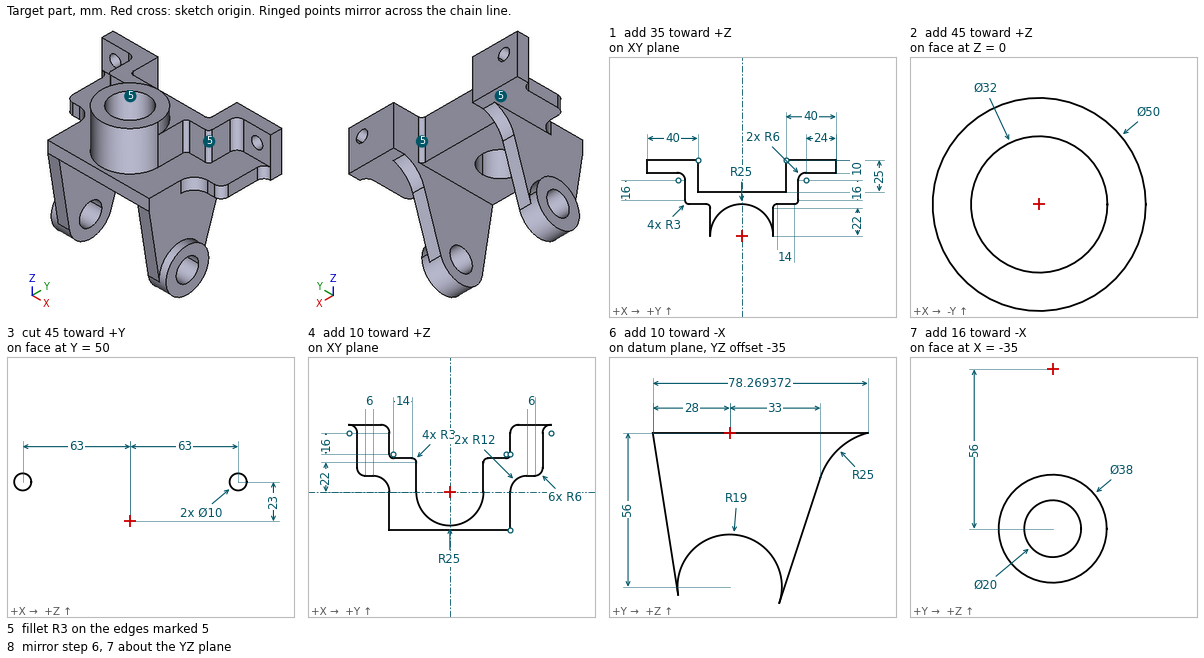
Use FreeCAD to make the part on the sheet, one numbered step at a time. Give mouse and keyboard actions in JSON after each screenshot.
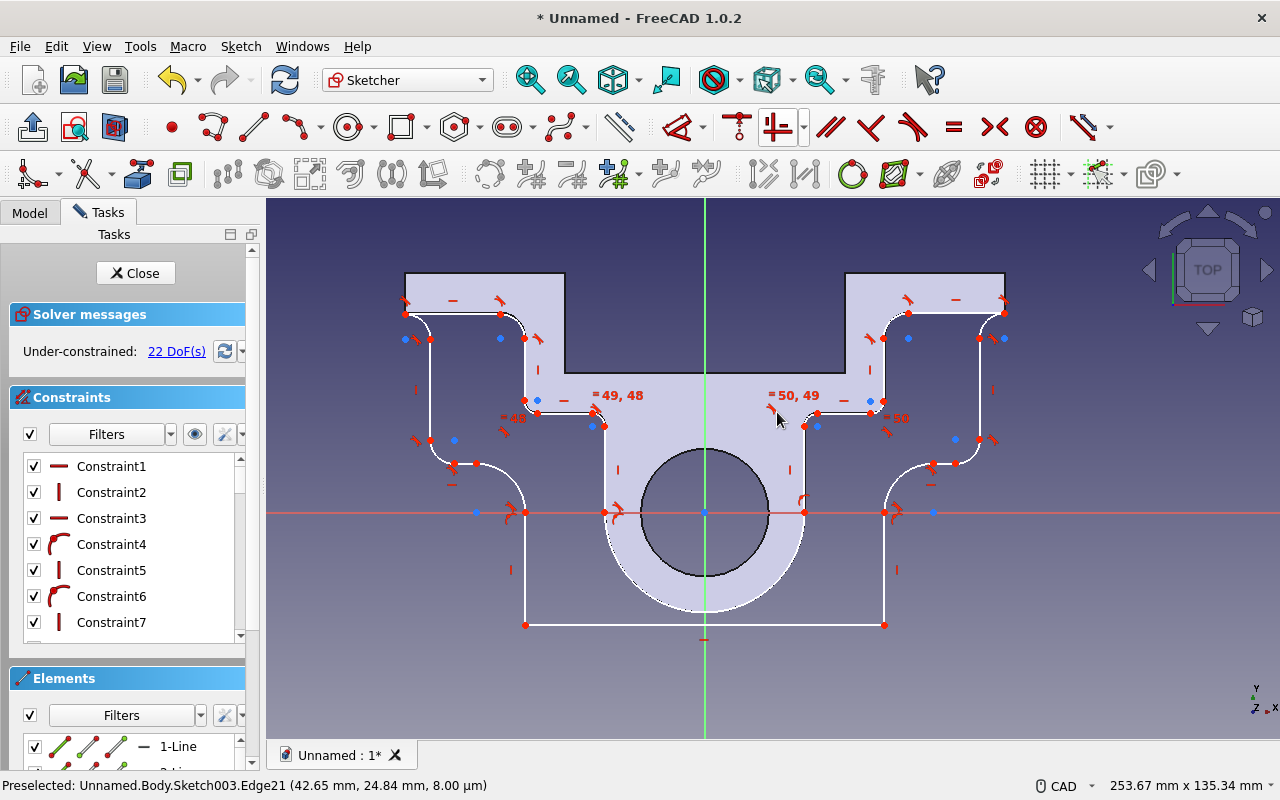
{"action": "scroll", "coordinate": [522, 327], "scroll_direction": "up", "scroll_amount": 2}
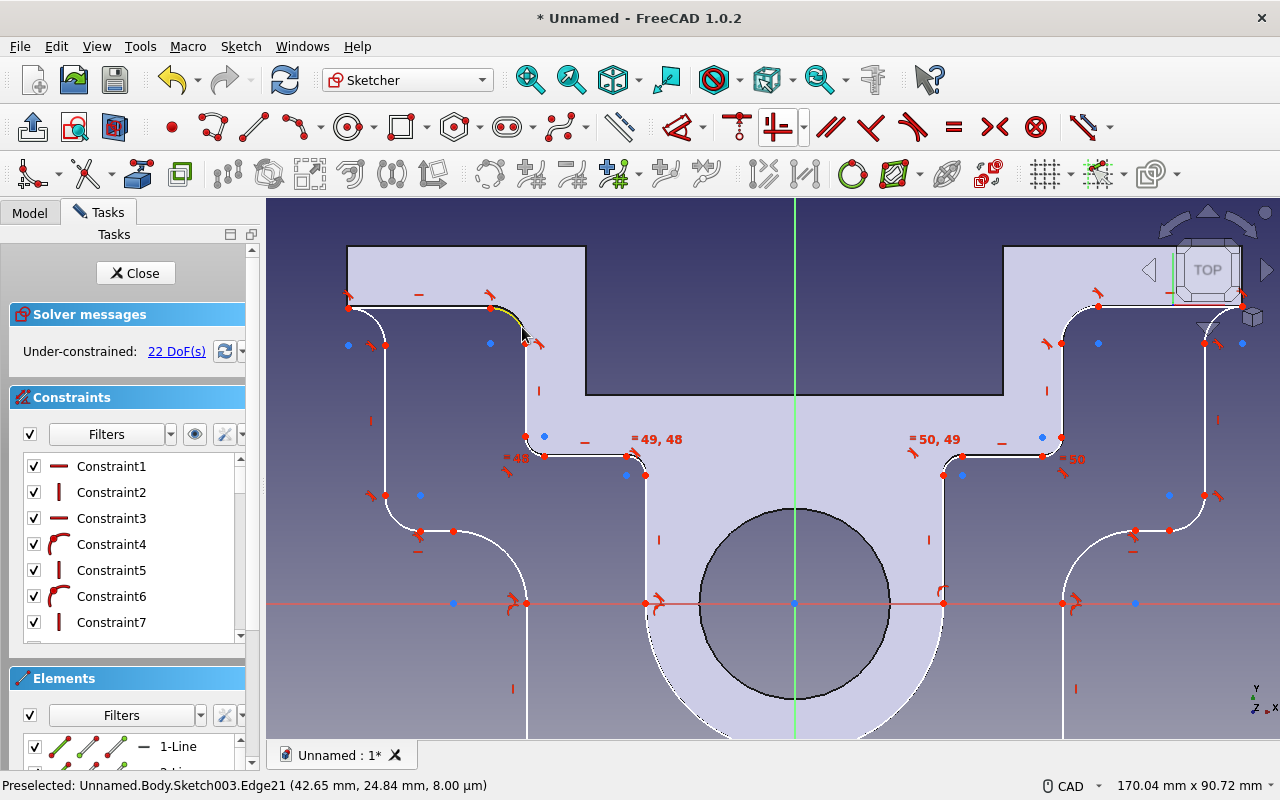
{"action": "left_click", "coordinate": [522, 328]}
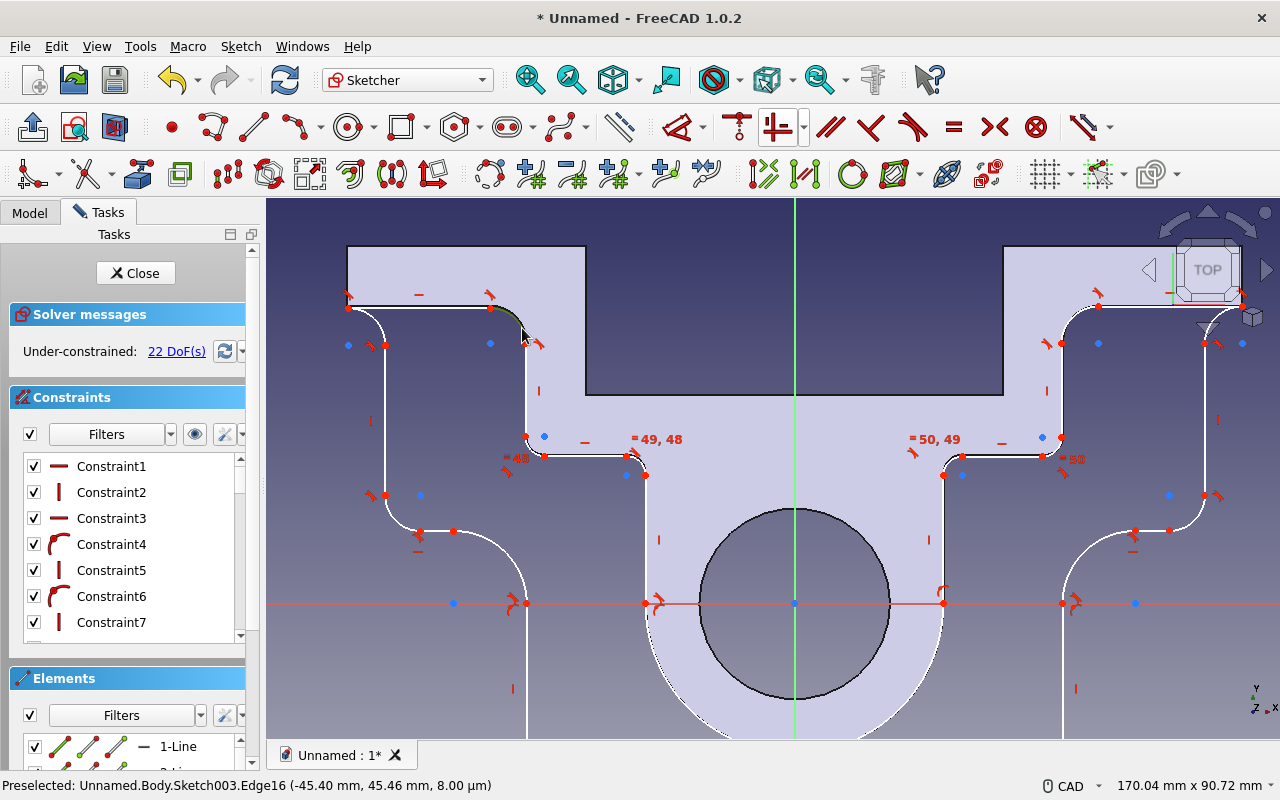
{"action": "left_click", "coordinate": [1082, 311]}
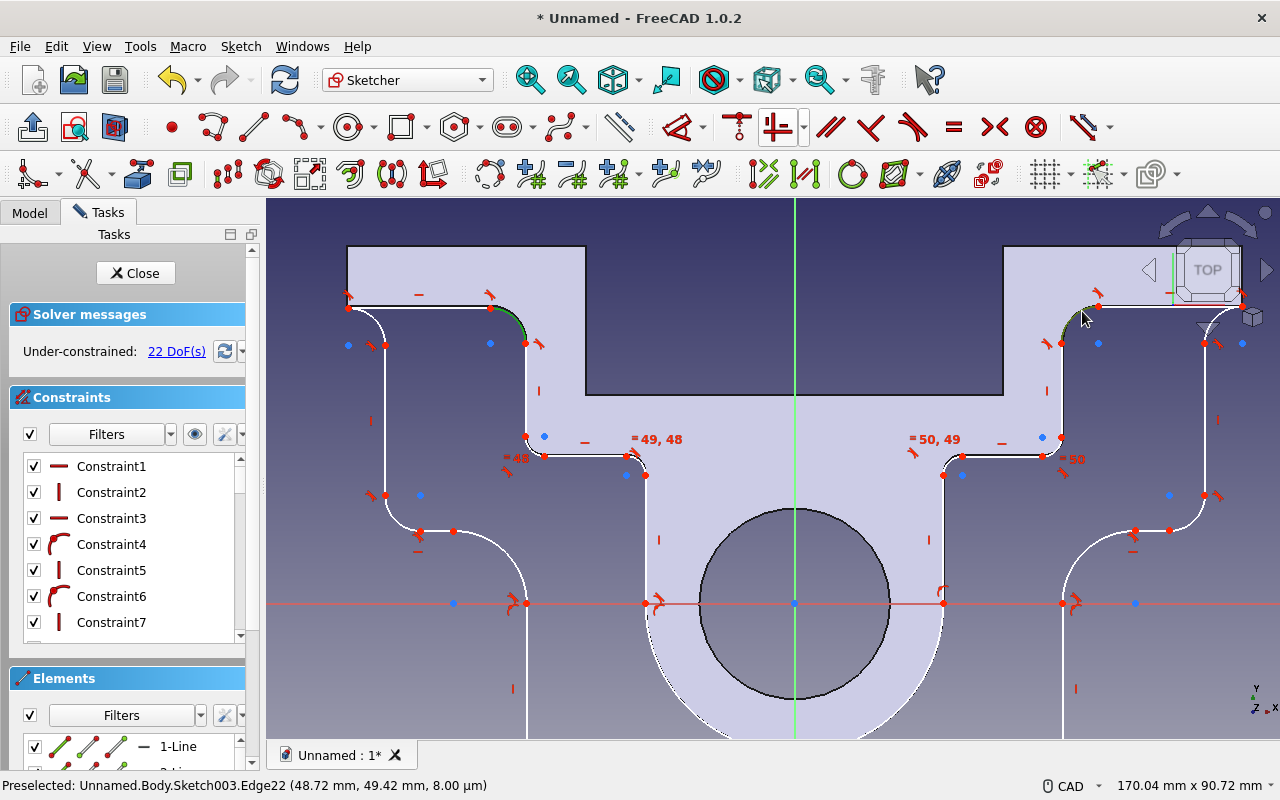
{"action": "scroll", "coordinate": [521, 327], "scroll_direction": "down", "scroll_amount": 2}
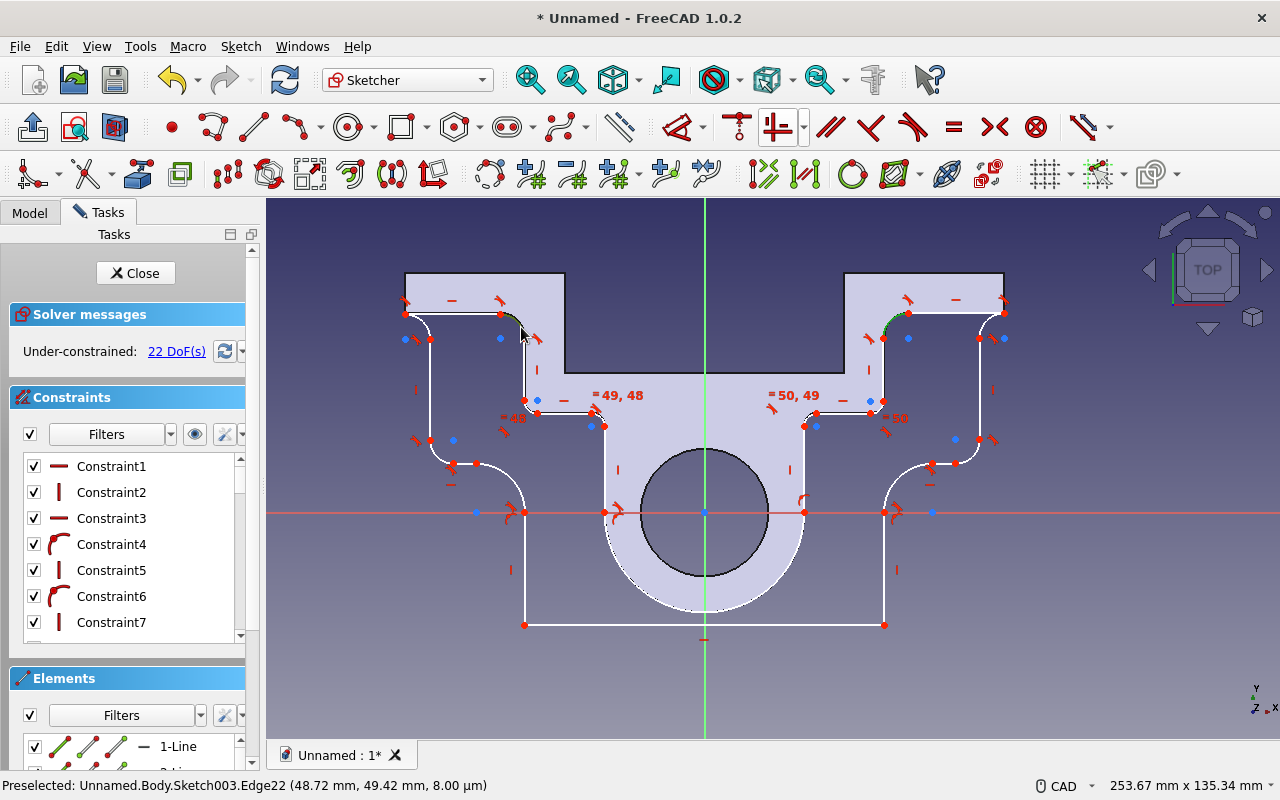
{"action": "left_click", "coordinate": [982, 327]}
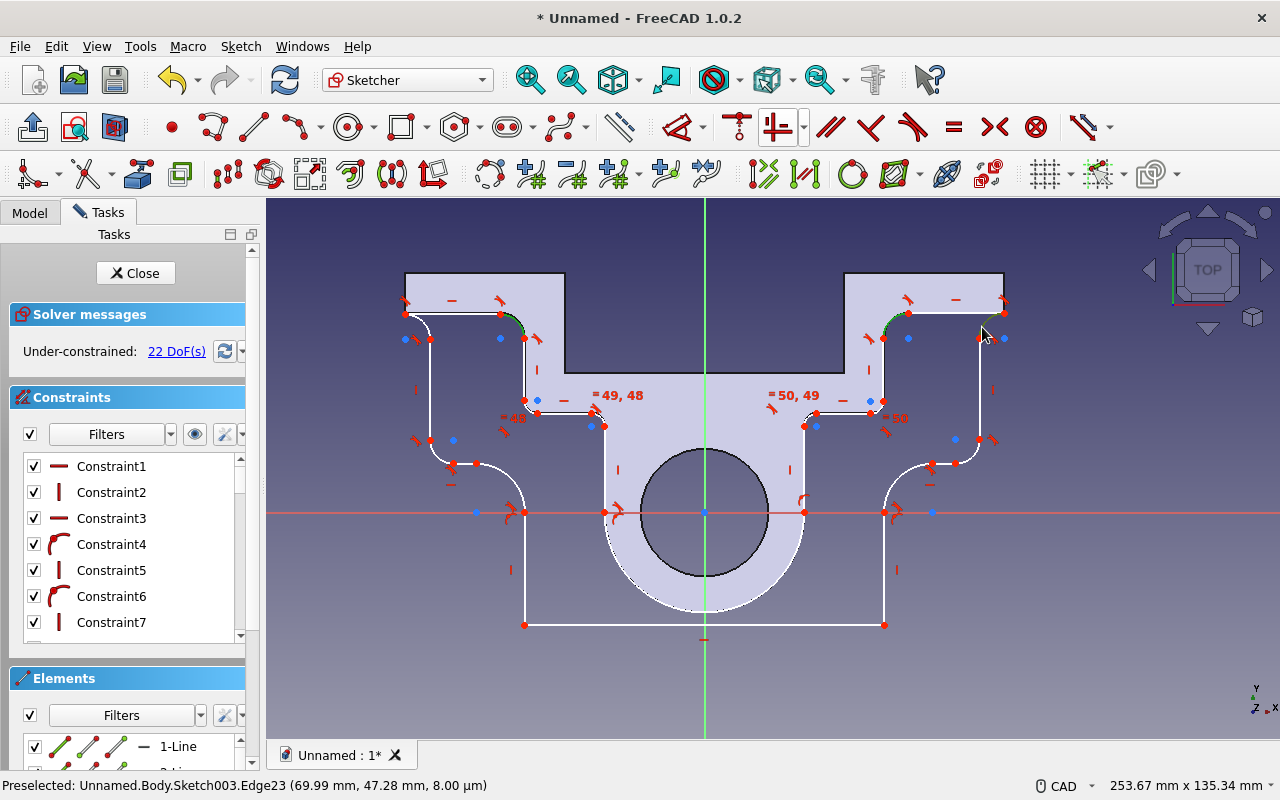
{"action": "scroll", "coordinate": [966, 461], "scroll_direction": "up", "scroll_amount": 2}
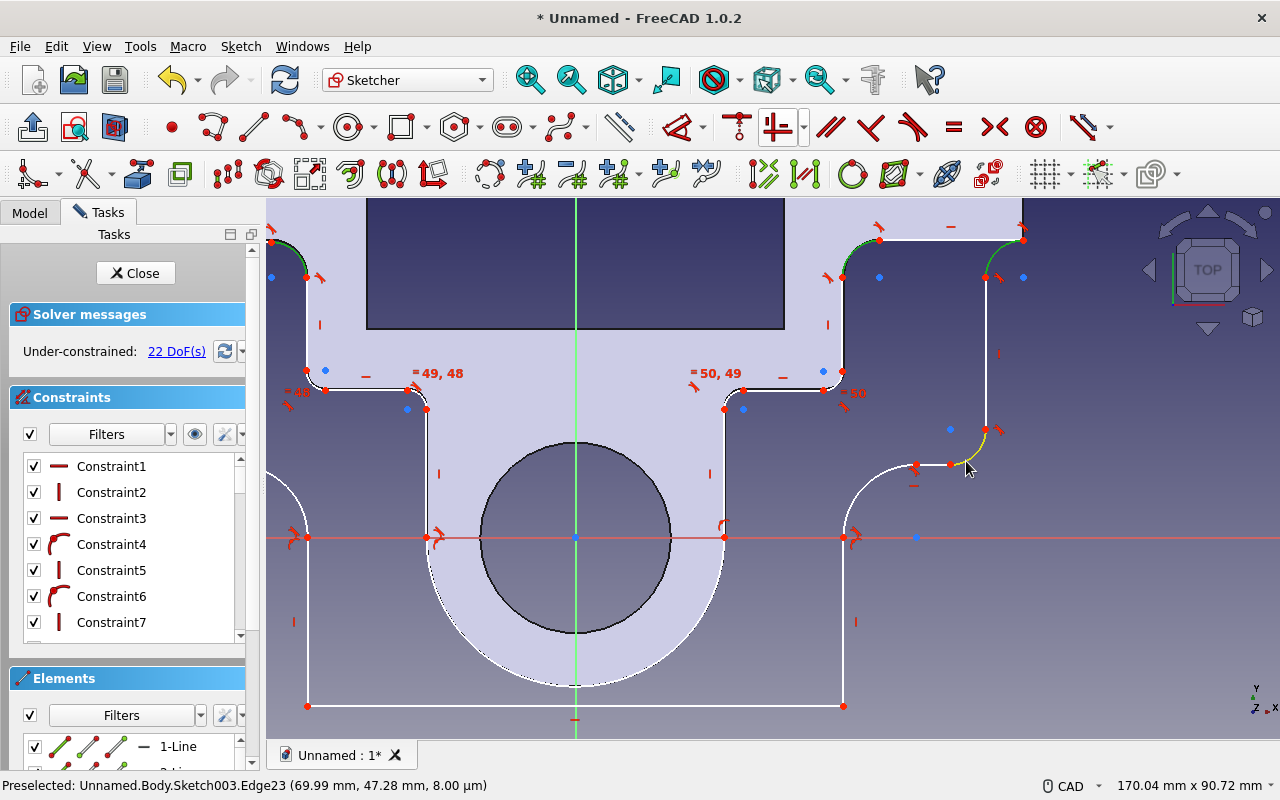
{"action": "left_click", "coordinate": [966, 461]}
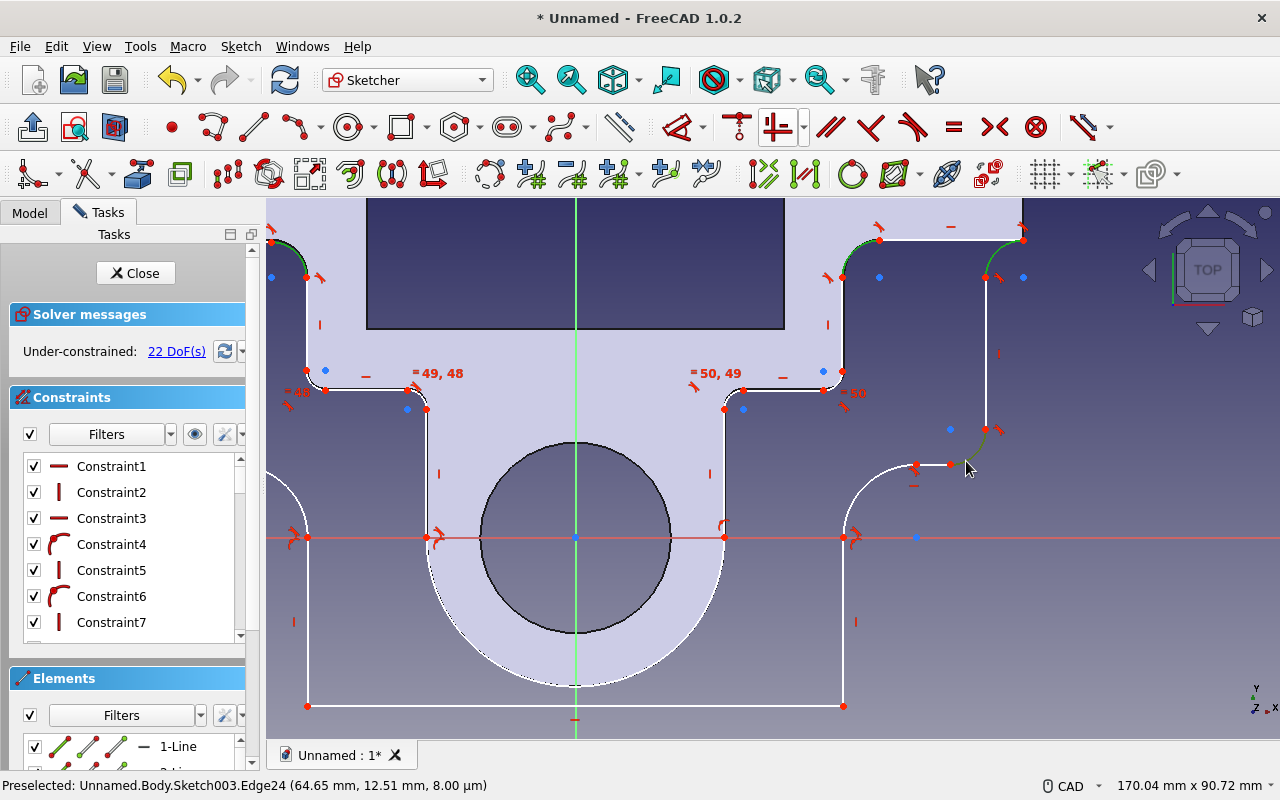
{"action": "scroll", "coordinate": [967, 461], "scroll_direction": "down", "scroll_amount": 2}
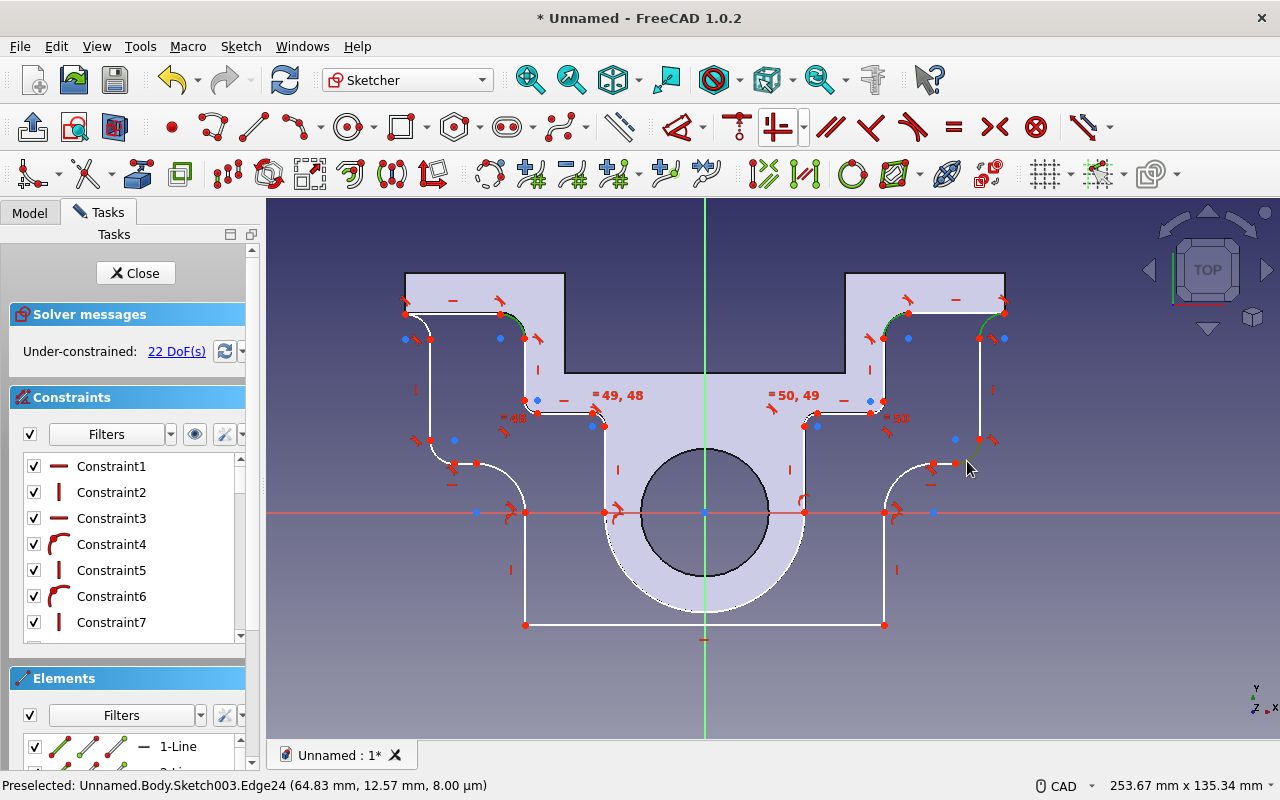
{"action": "scroll", "coordinate": [433, 451], "scroll_direction": "up", "scroll_amount": 2}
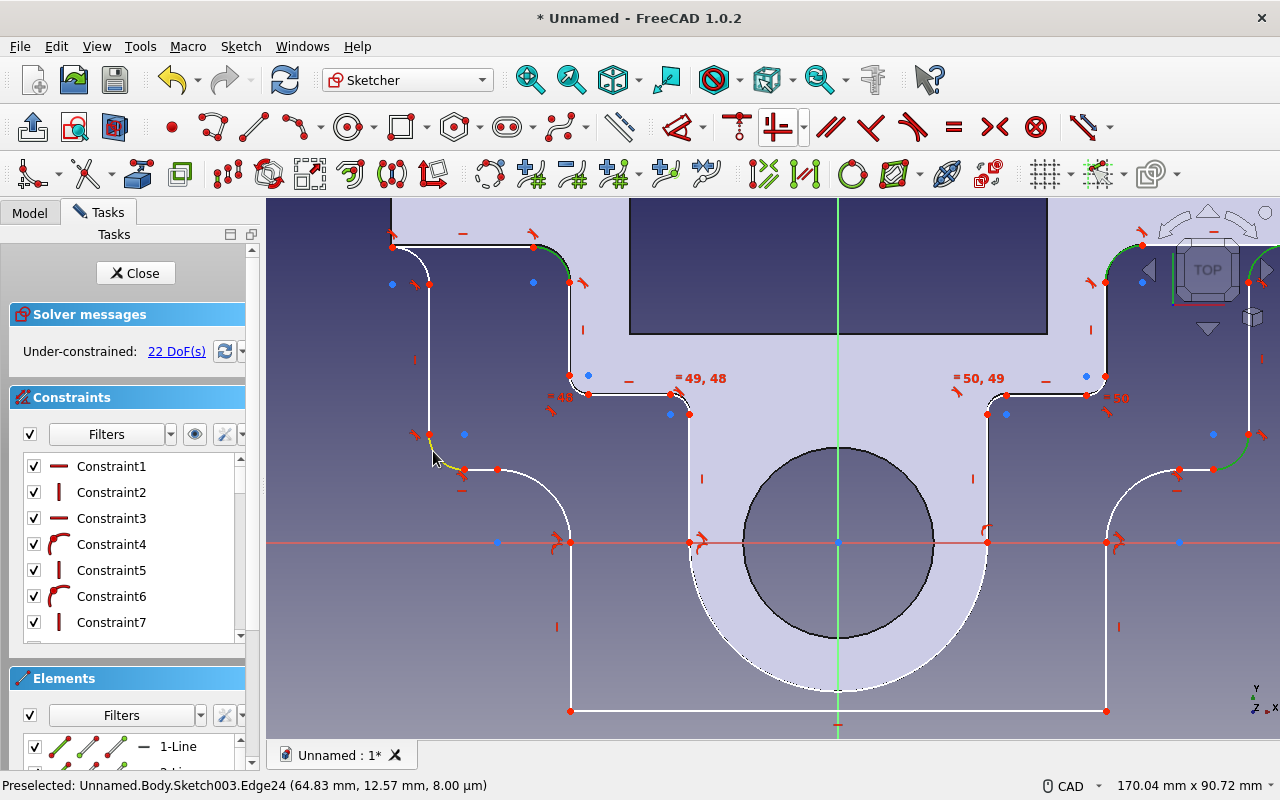
{"action": "left_click", "coordinate": [433, 451]}